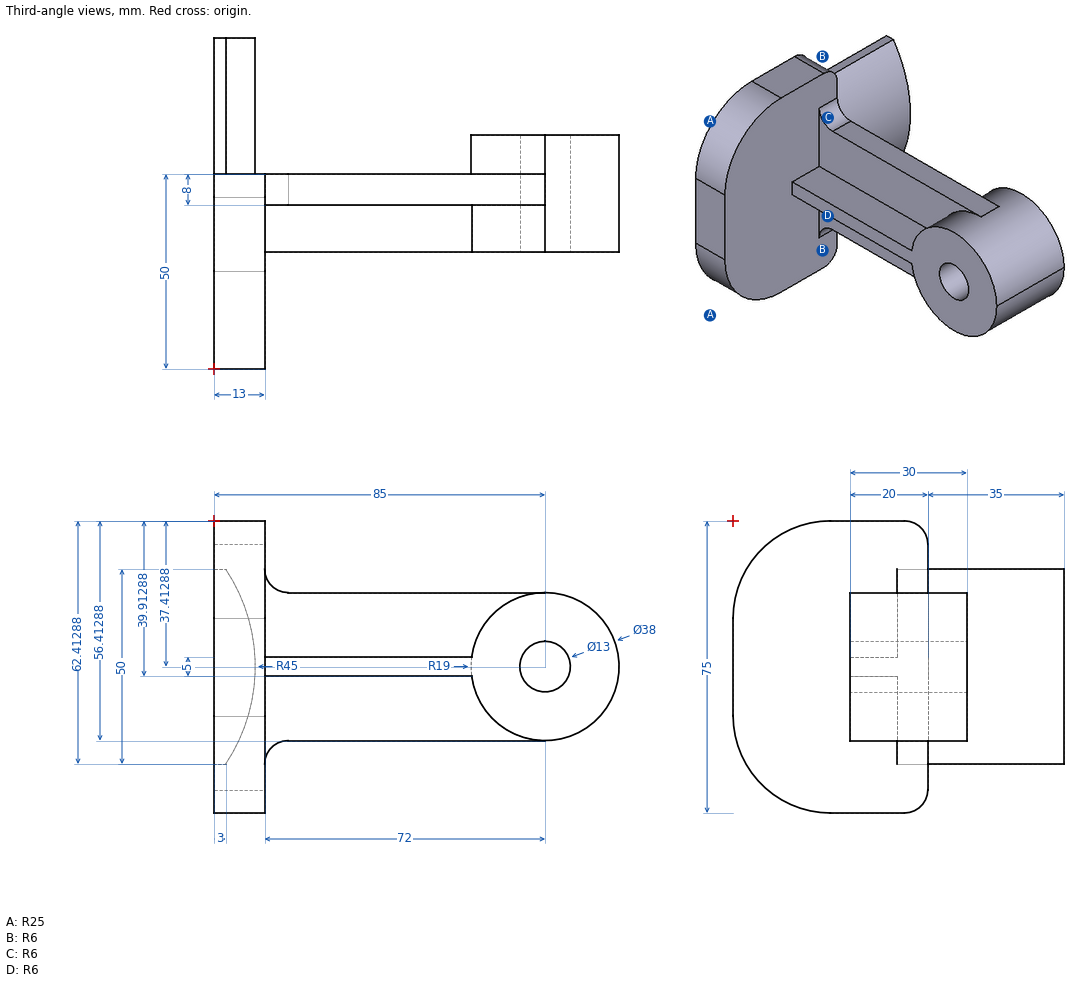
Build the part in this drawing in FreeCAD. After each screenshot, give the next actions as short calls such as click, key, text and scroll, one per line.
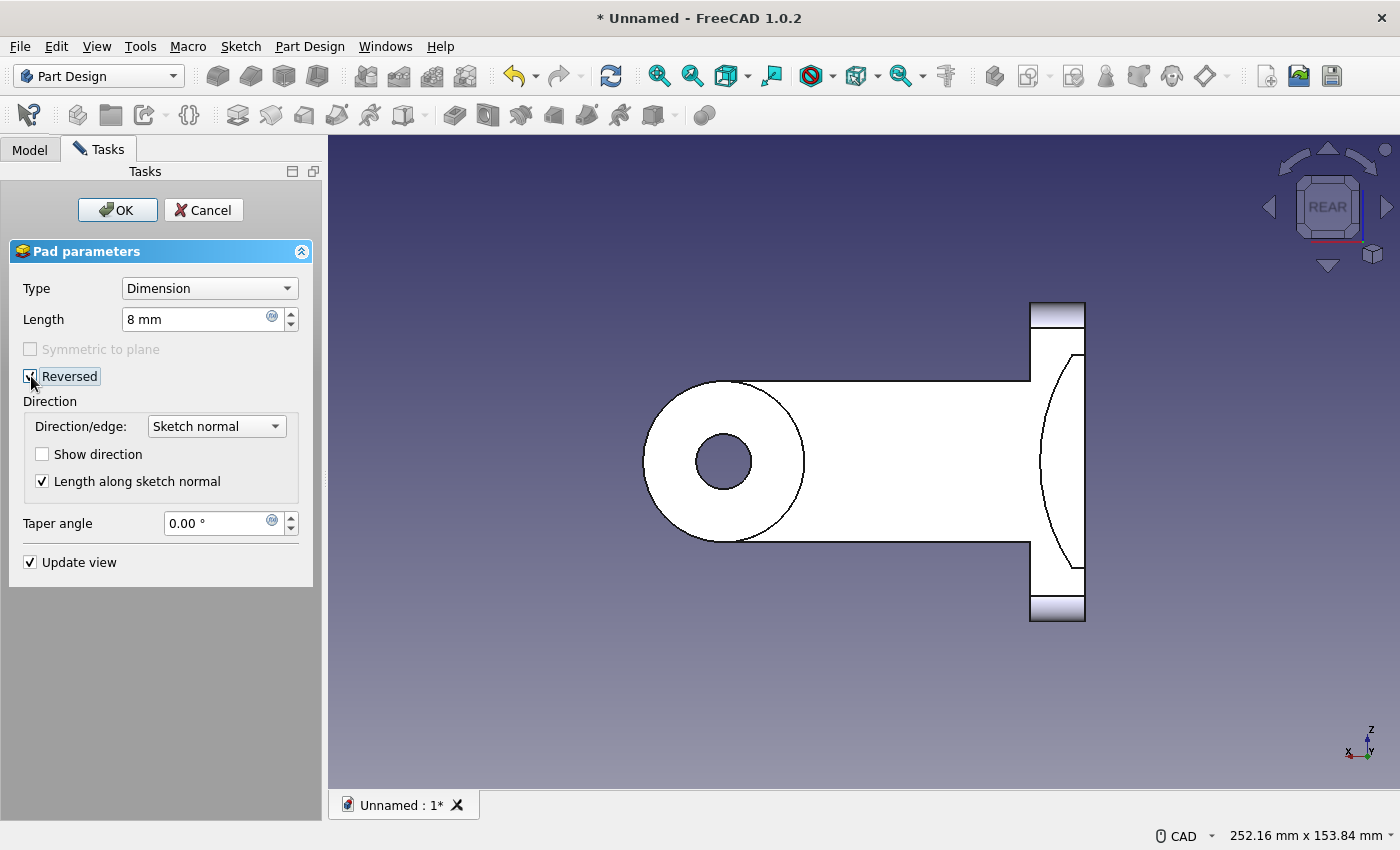
click(118, 210)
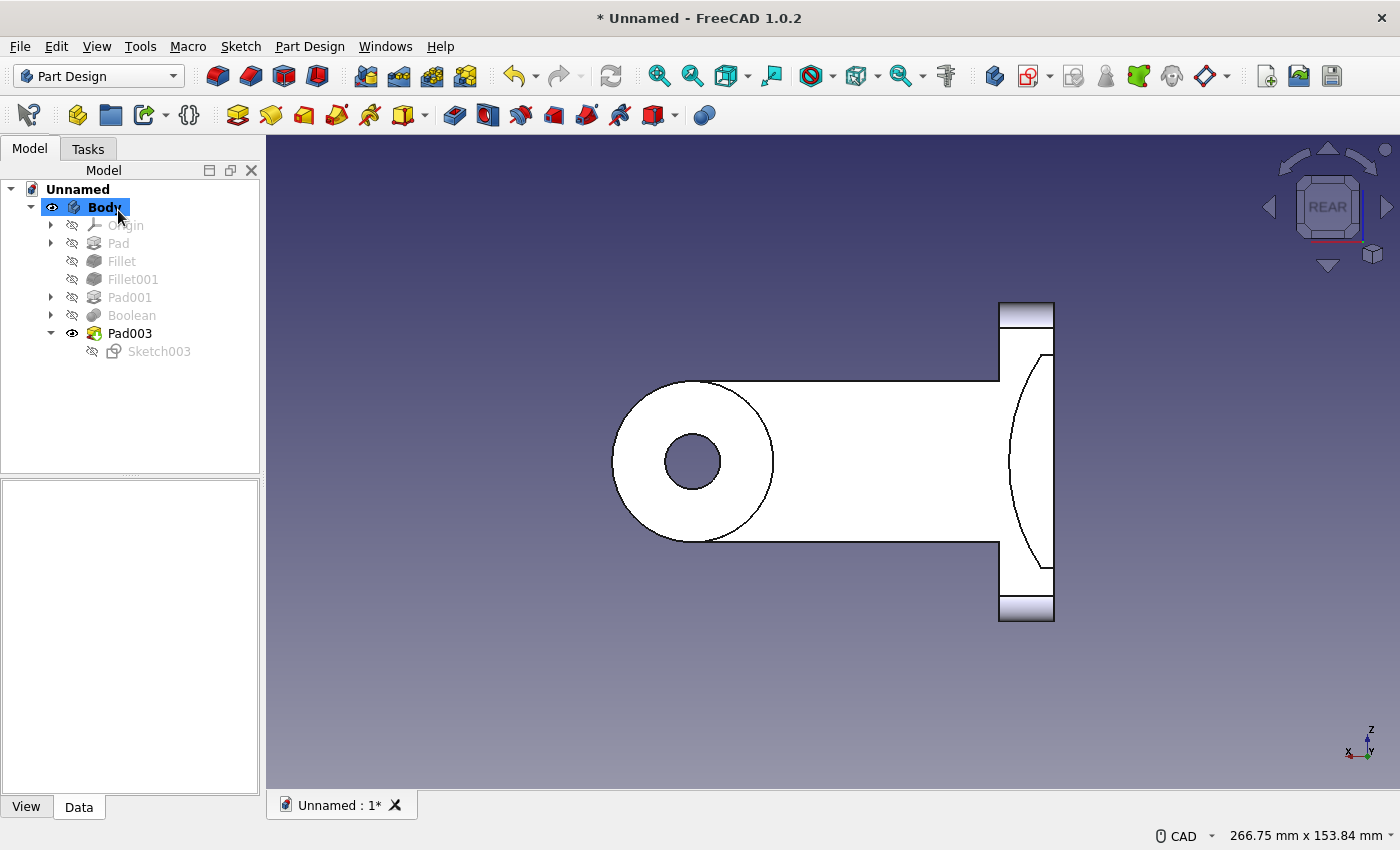
key(0)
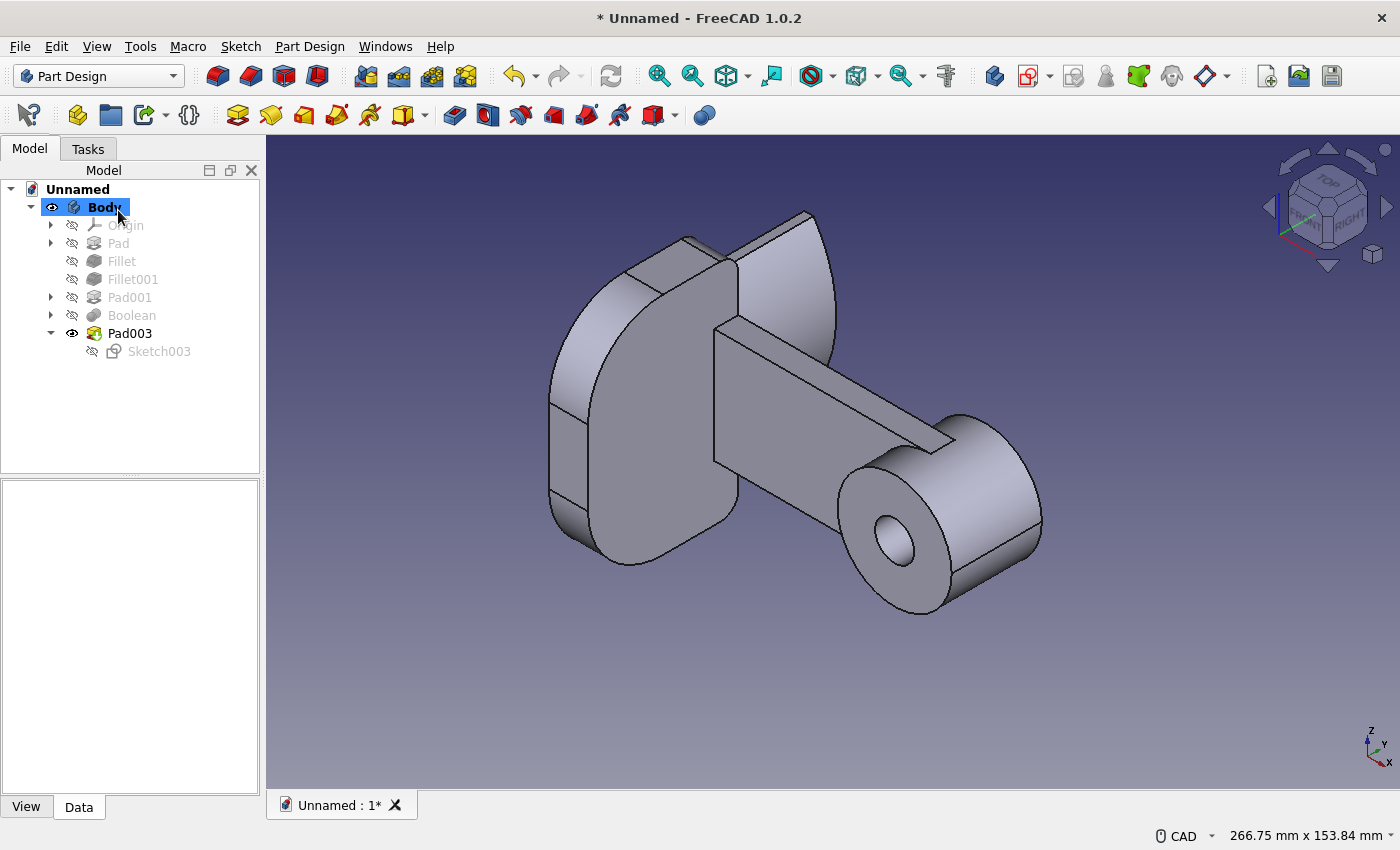
click(927, 540)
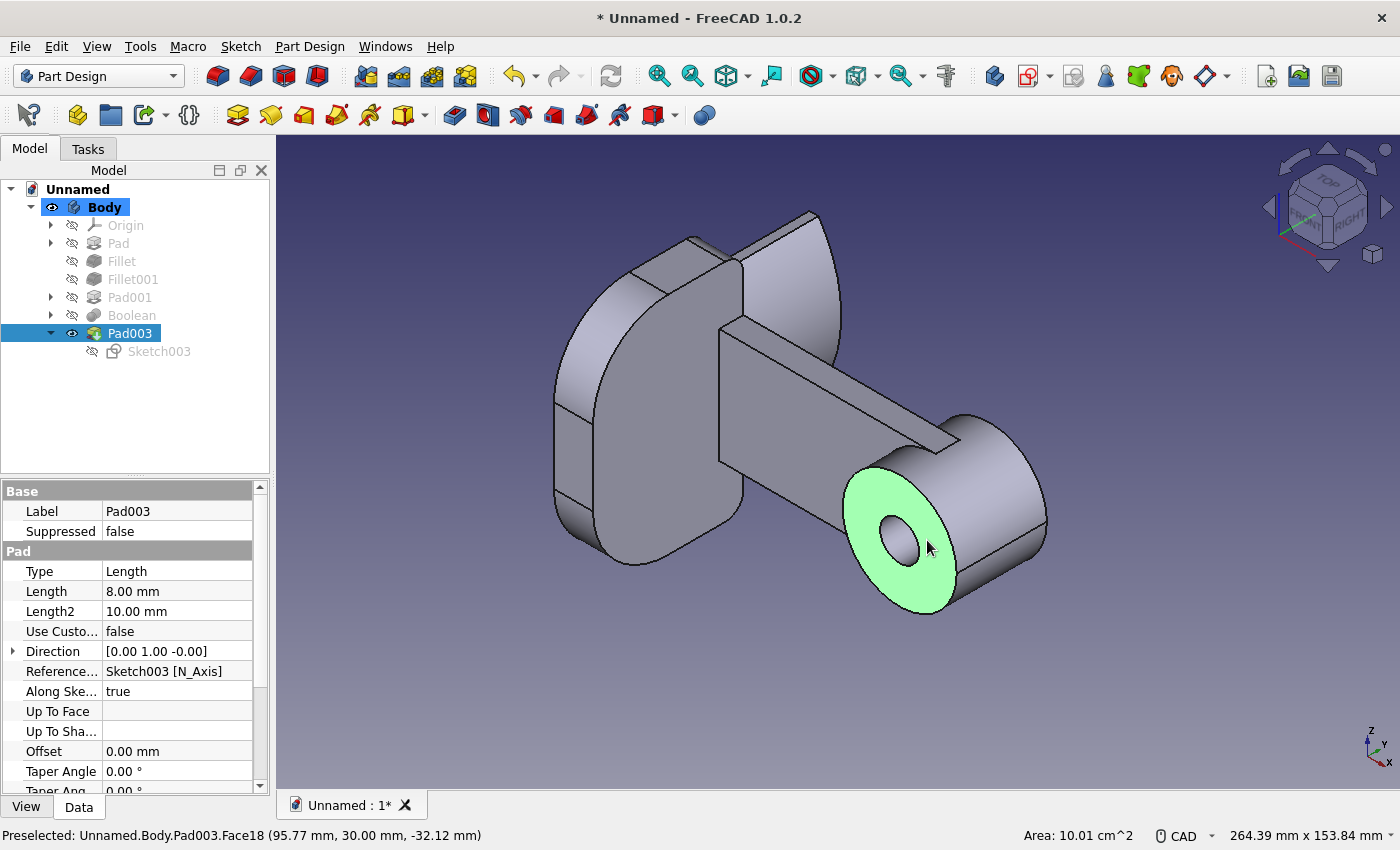
click(1028, 76)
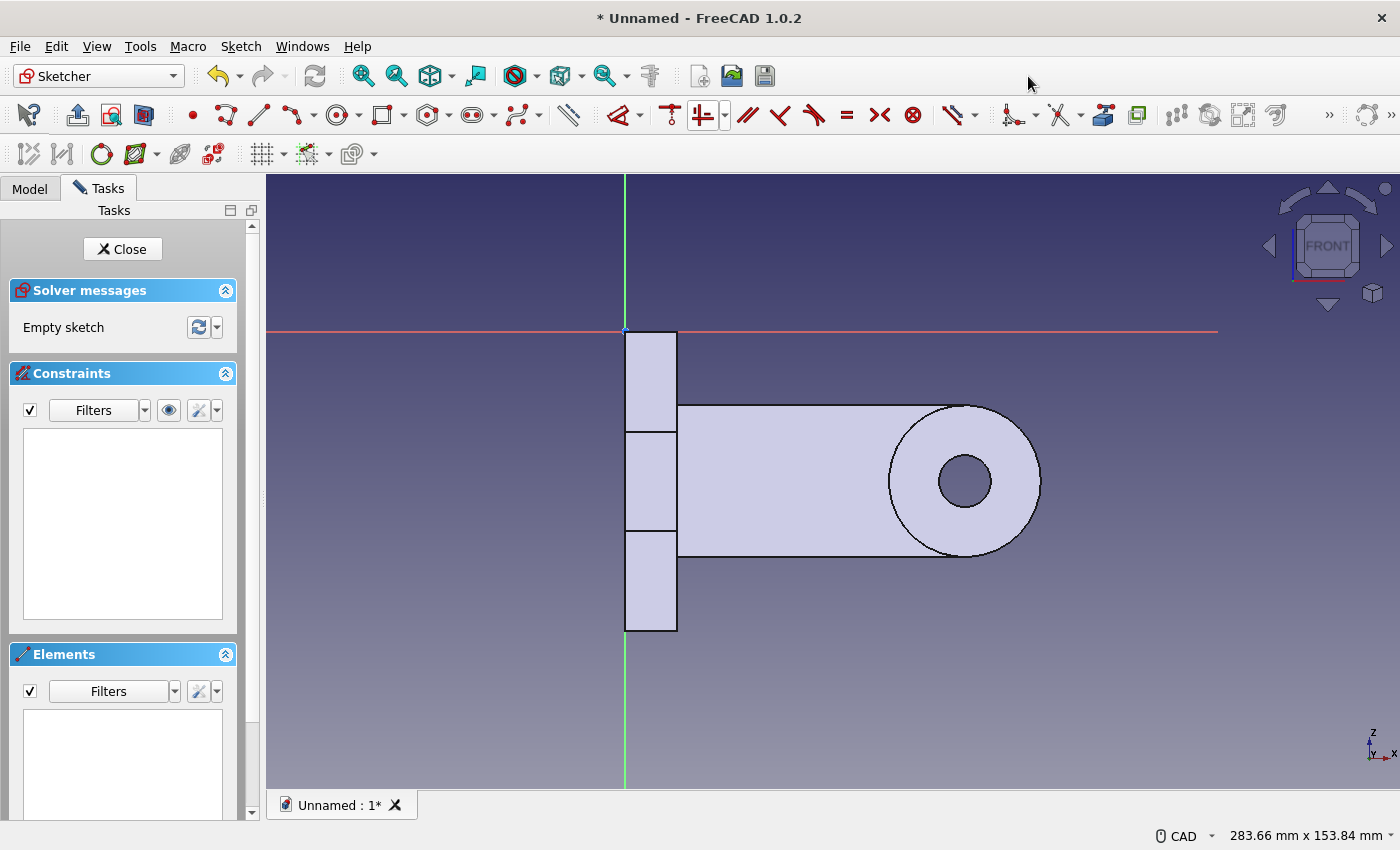
scroll(753, 371, up, 5)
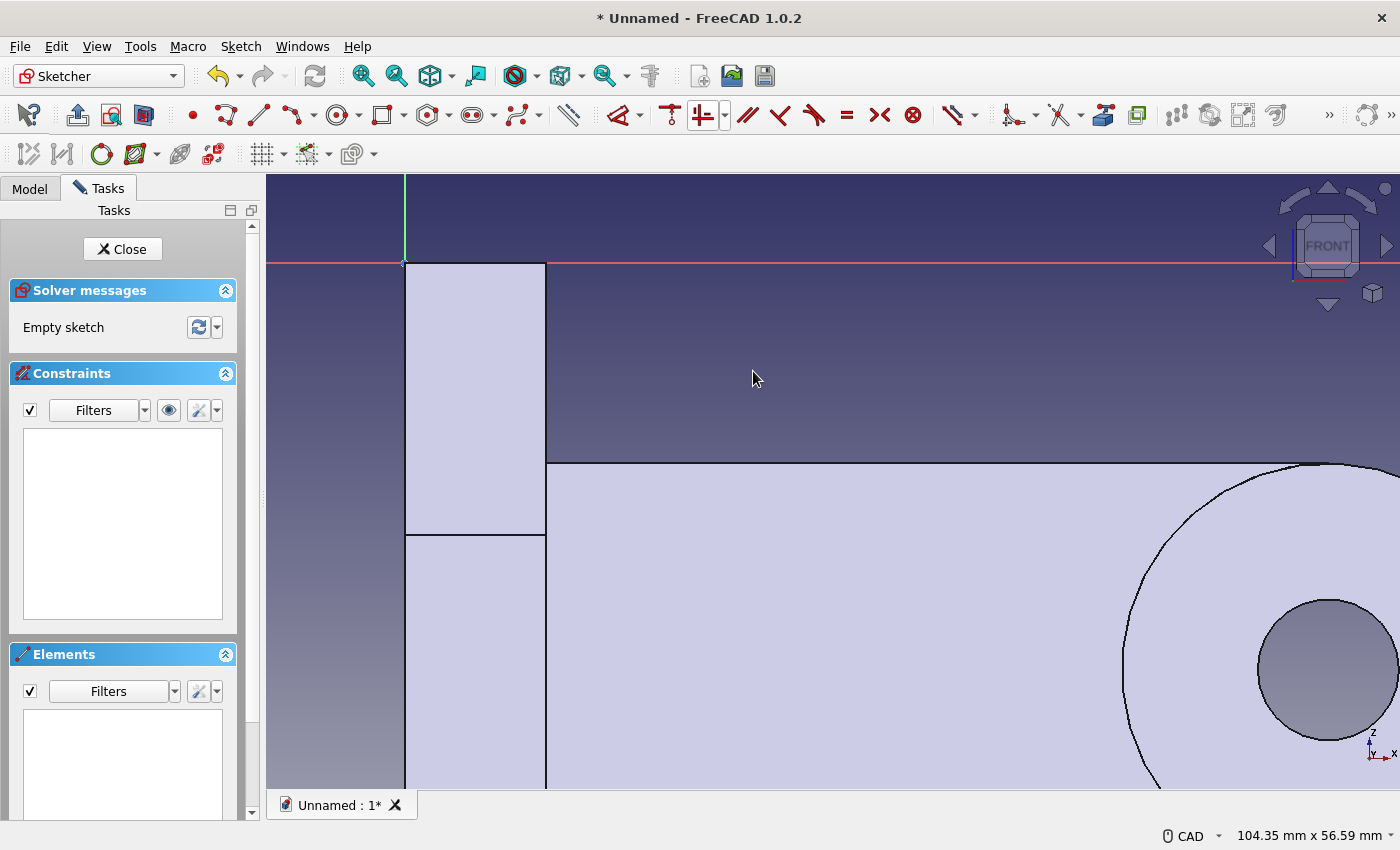
click(226, 116)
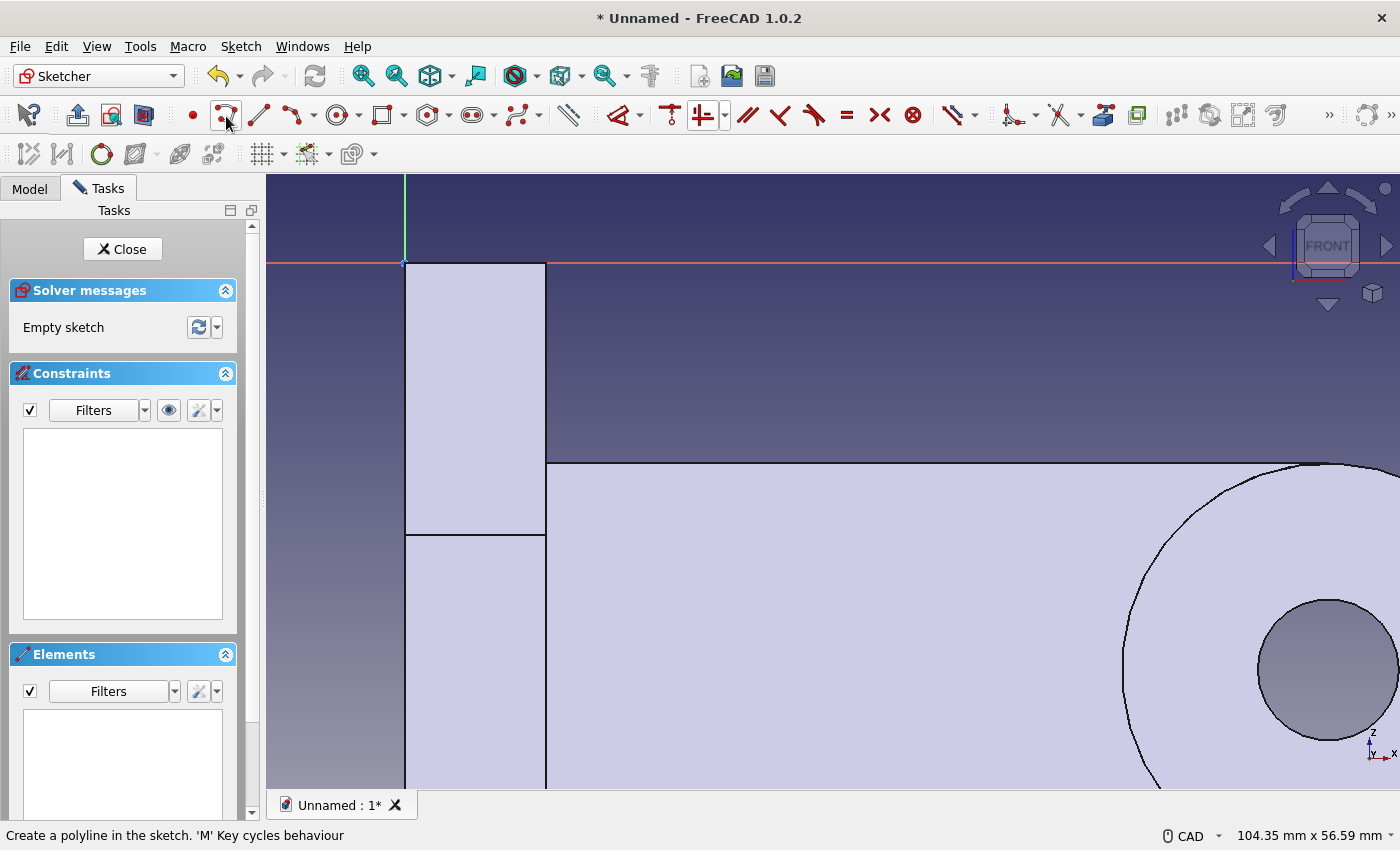
click(1124, 697)
click(405, 697)
click(414, 643)
click(1124, 643)
right_click(1124, 643)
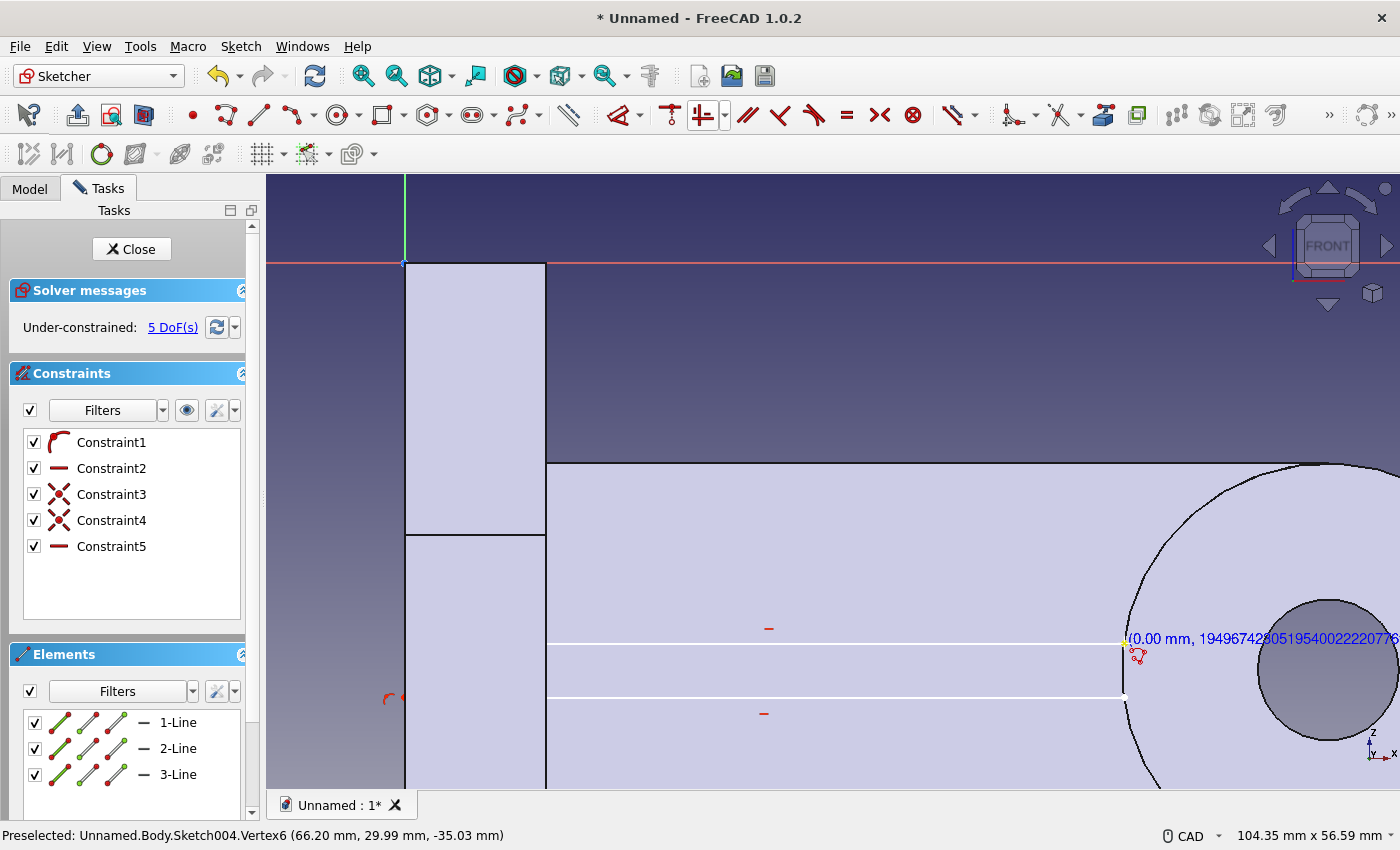
click(292, 116)